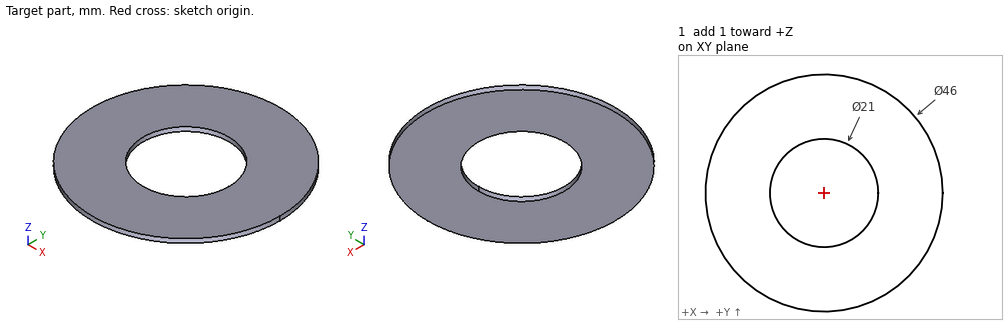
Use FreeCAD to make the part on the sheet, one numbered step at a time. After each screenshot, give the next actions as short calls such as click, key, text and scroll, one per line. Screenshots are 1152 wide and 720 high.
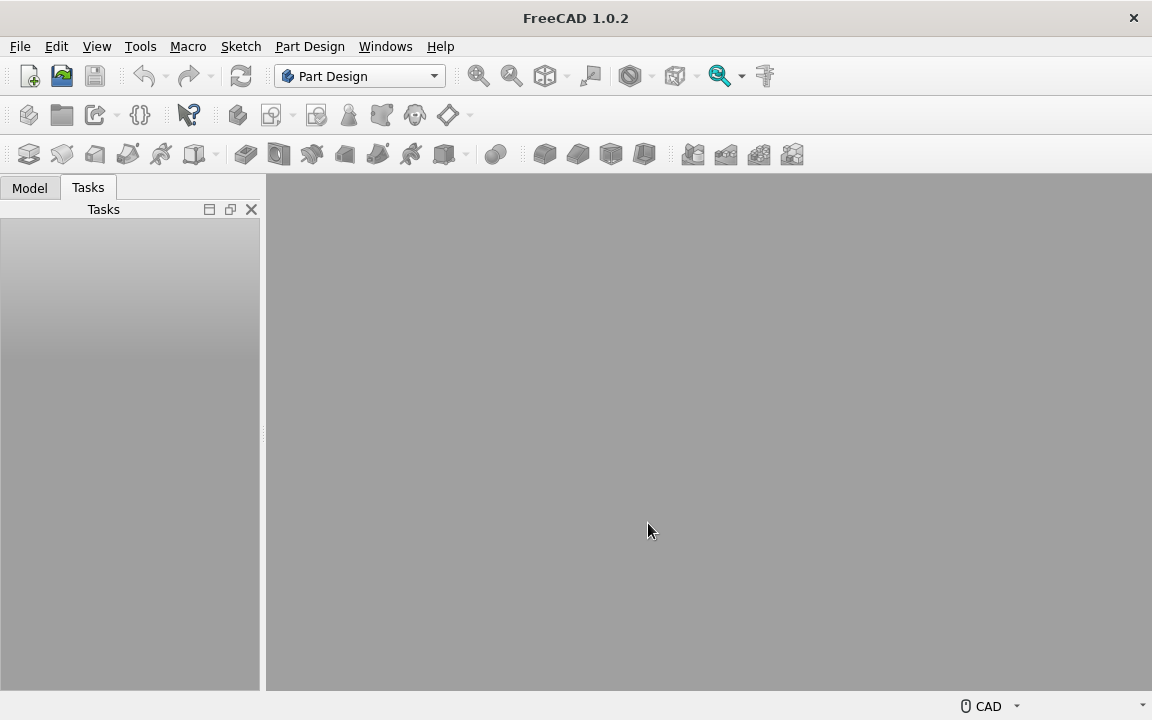
key(ctrl+n)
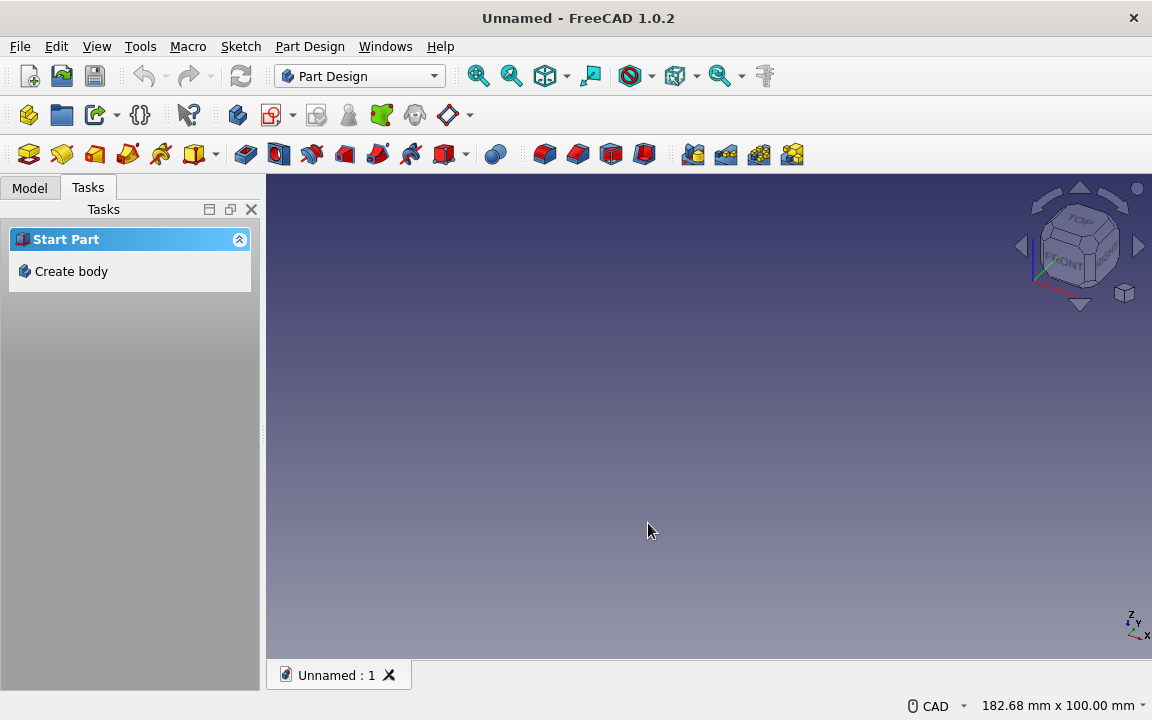
click(270, 116)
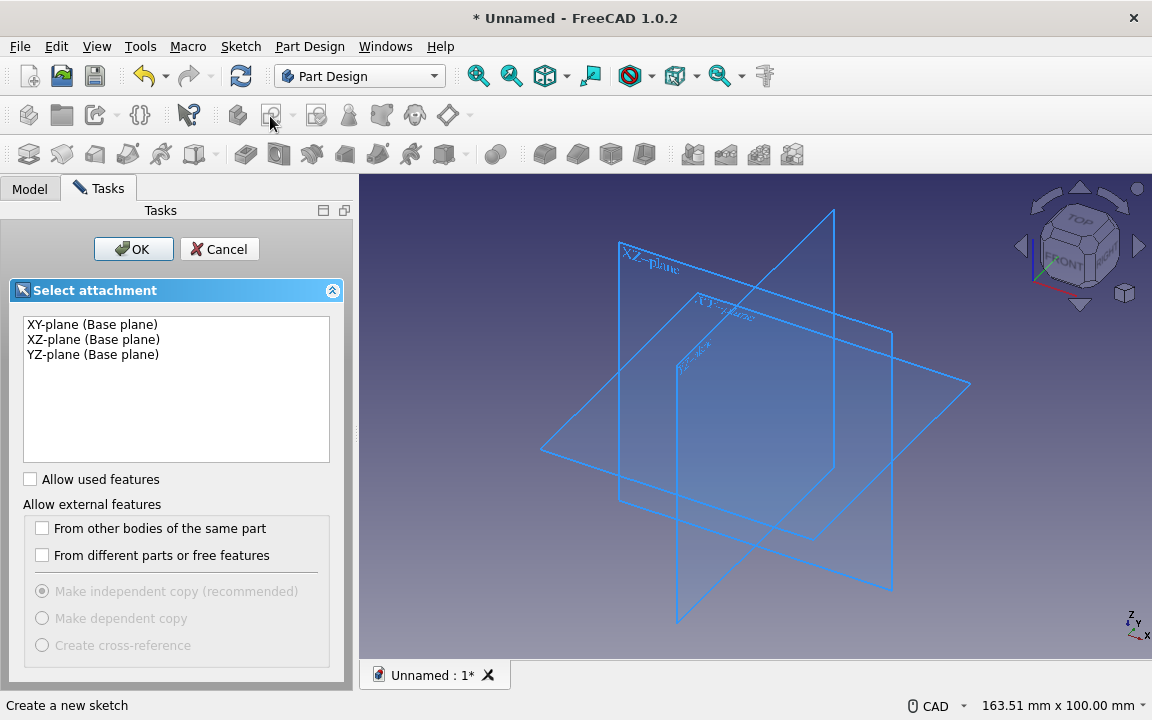
click(84, 324)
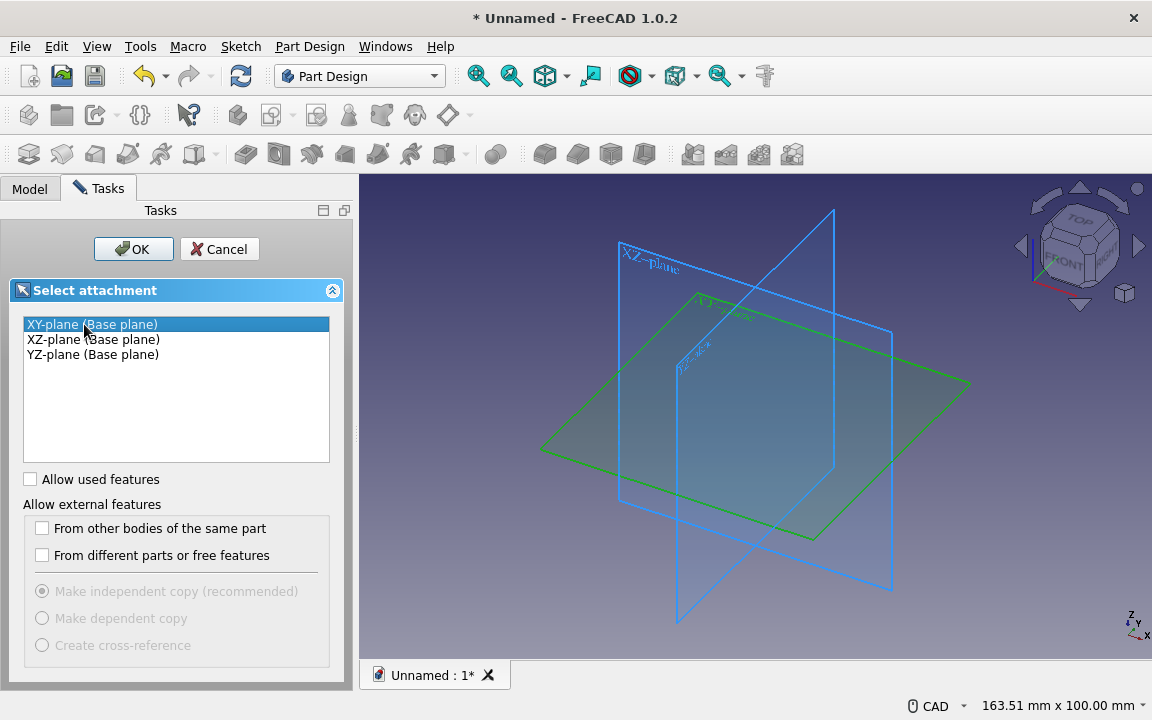
click(134, 249)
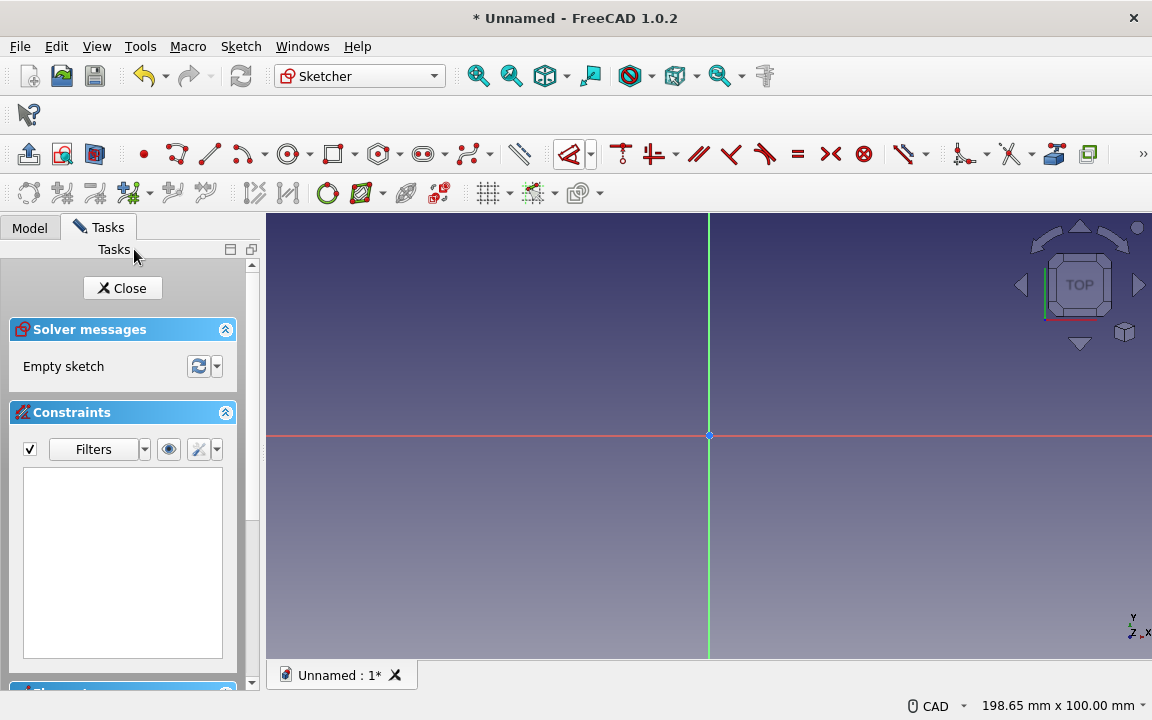
key(g)
key(c)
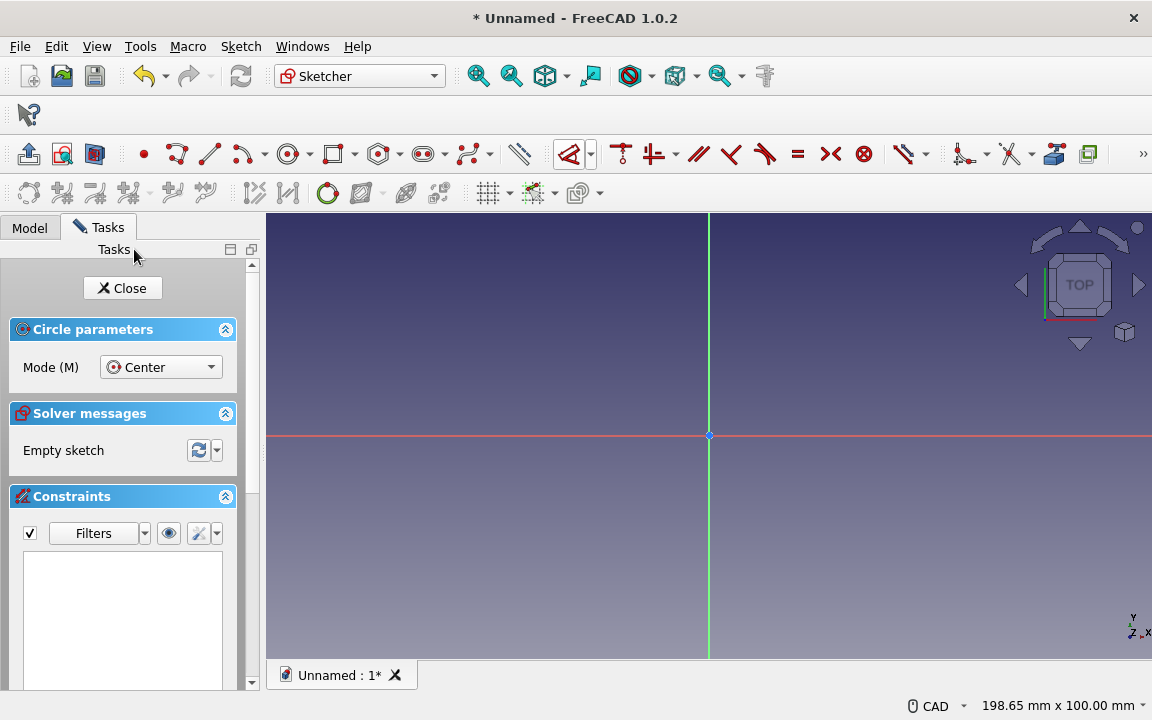
click(709, 436)
click(782, 363)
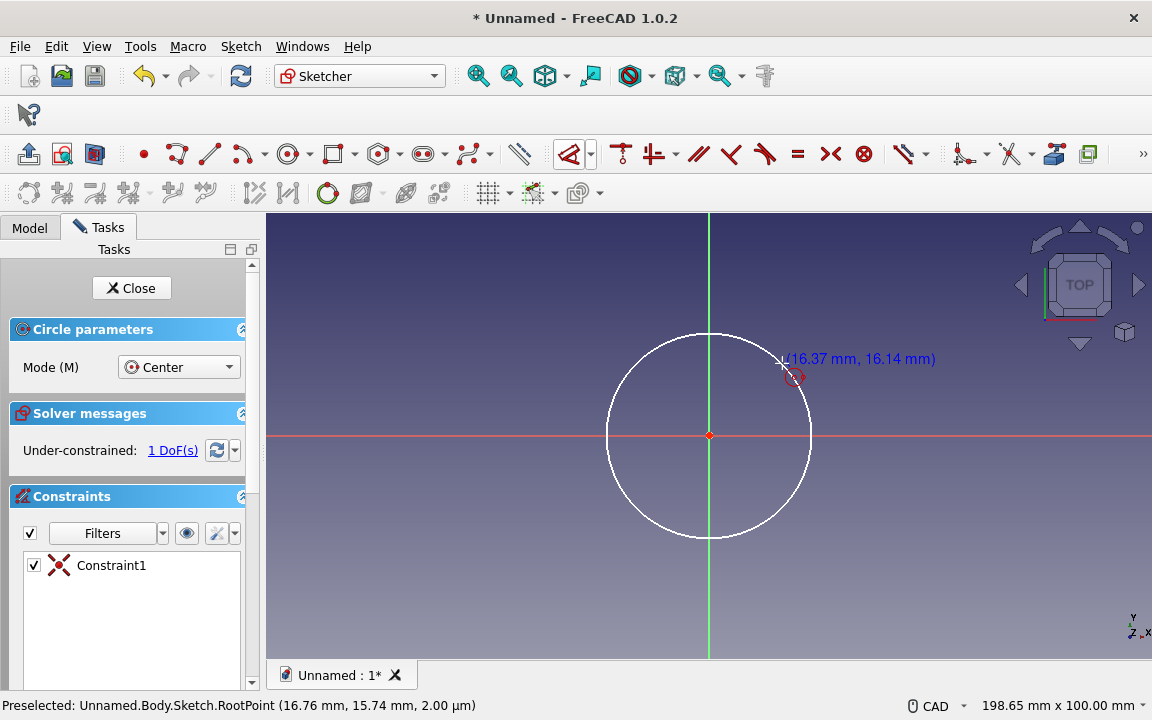
click(709, 436)
click(742, 403)
key(Escape)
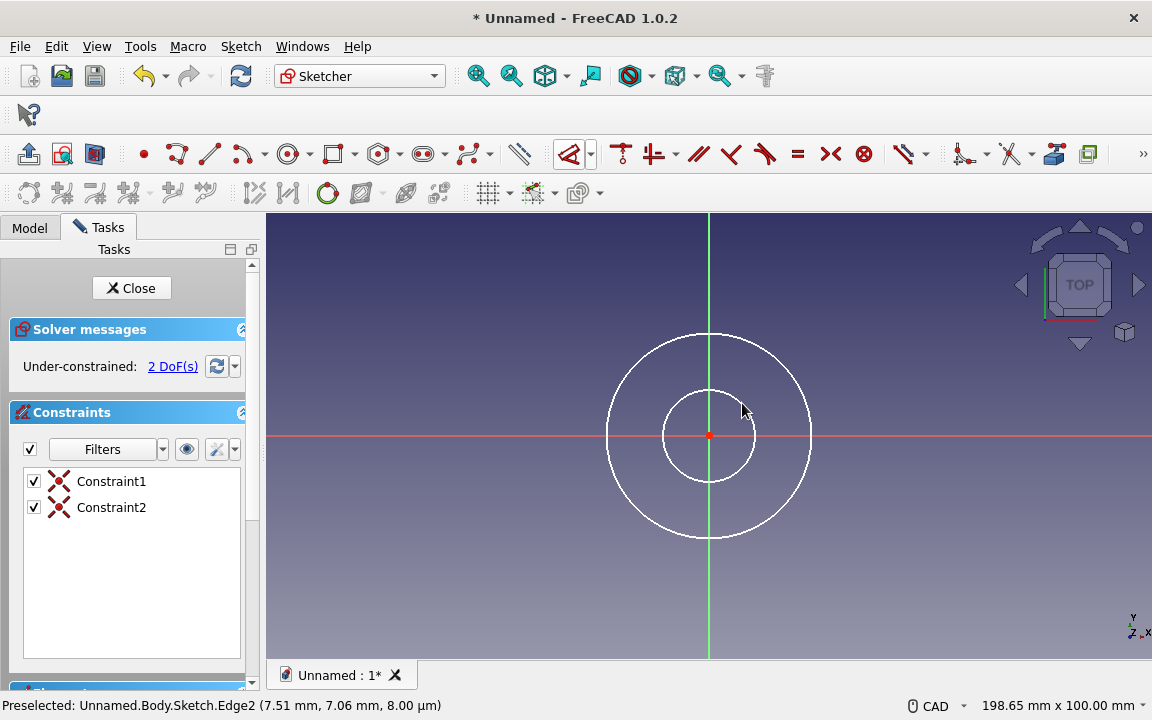
key(d)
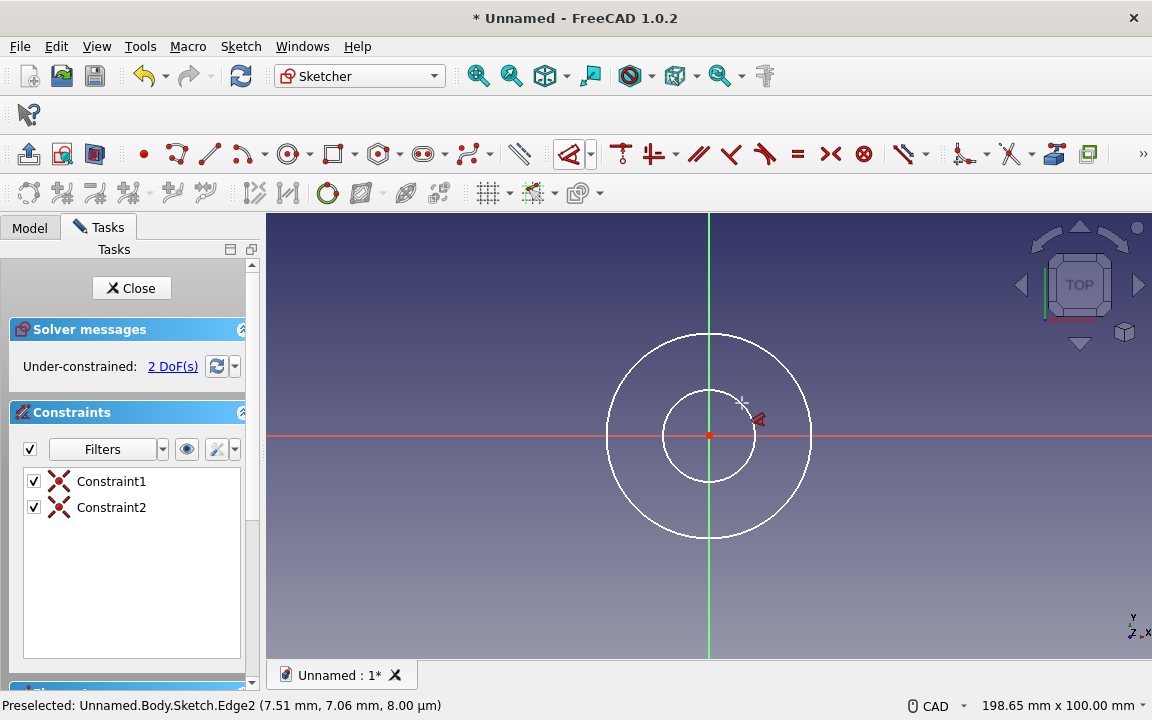
click(781, 363)
click(803, 340)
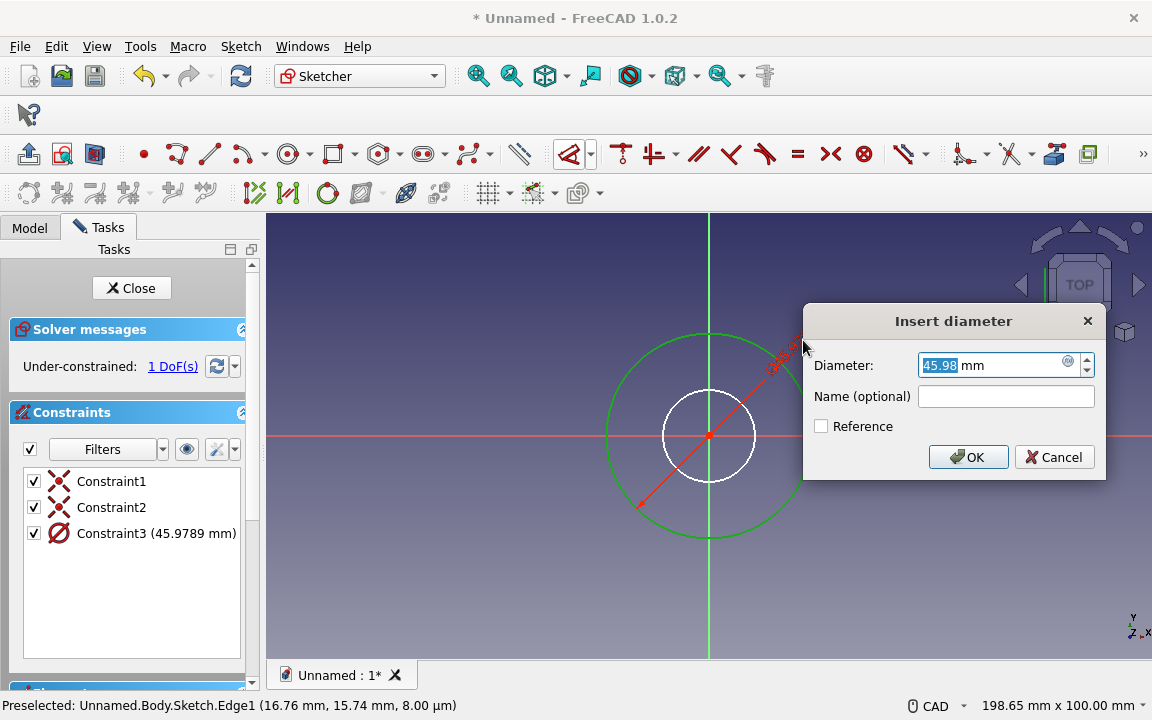
text(46)
key(Return)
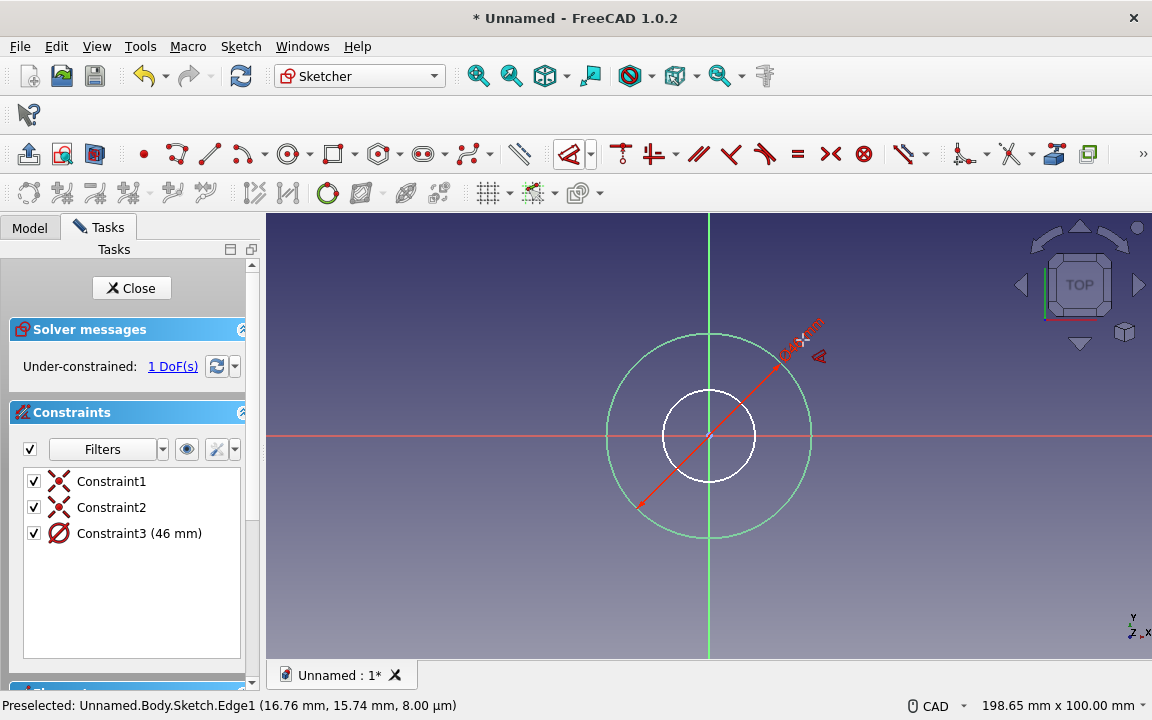
click(741, 403)
click(763, 380)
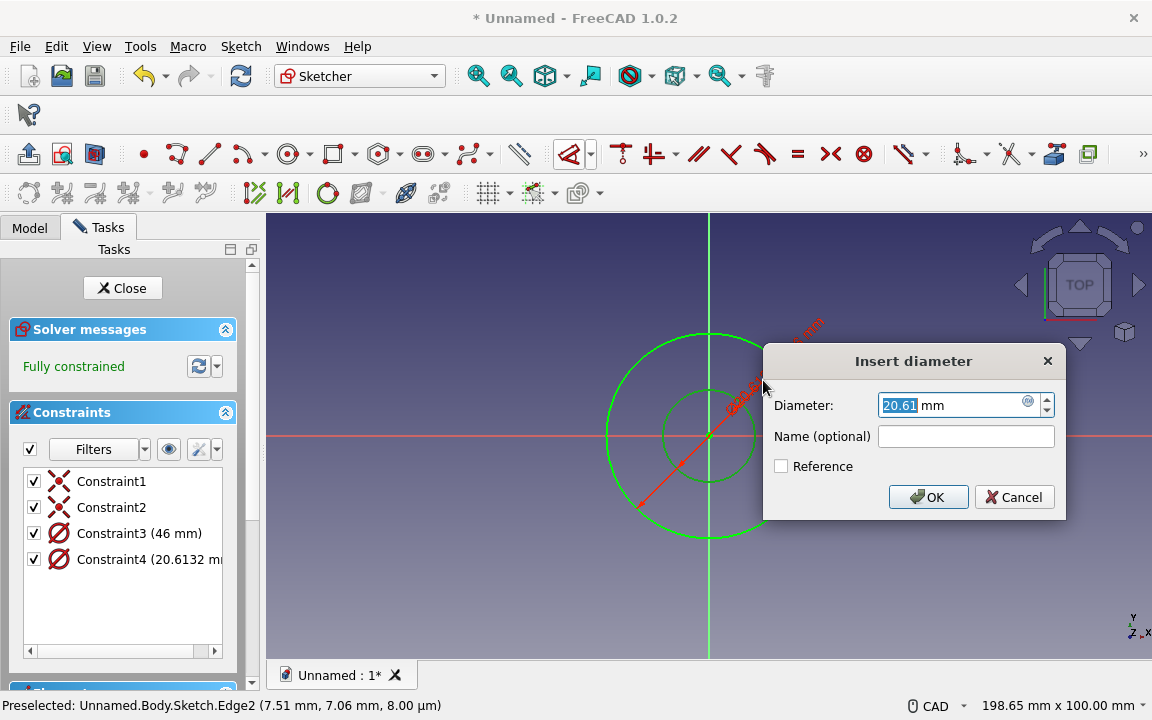
text(21)
key(Return)
key(Escape)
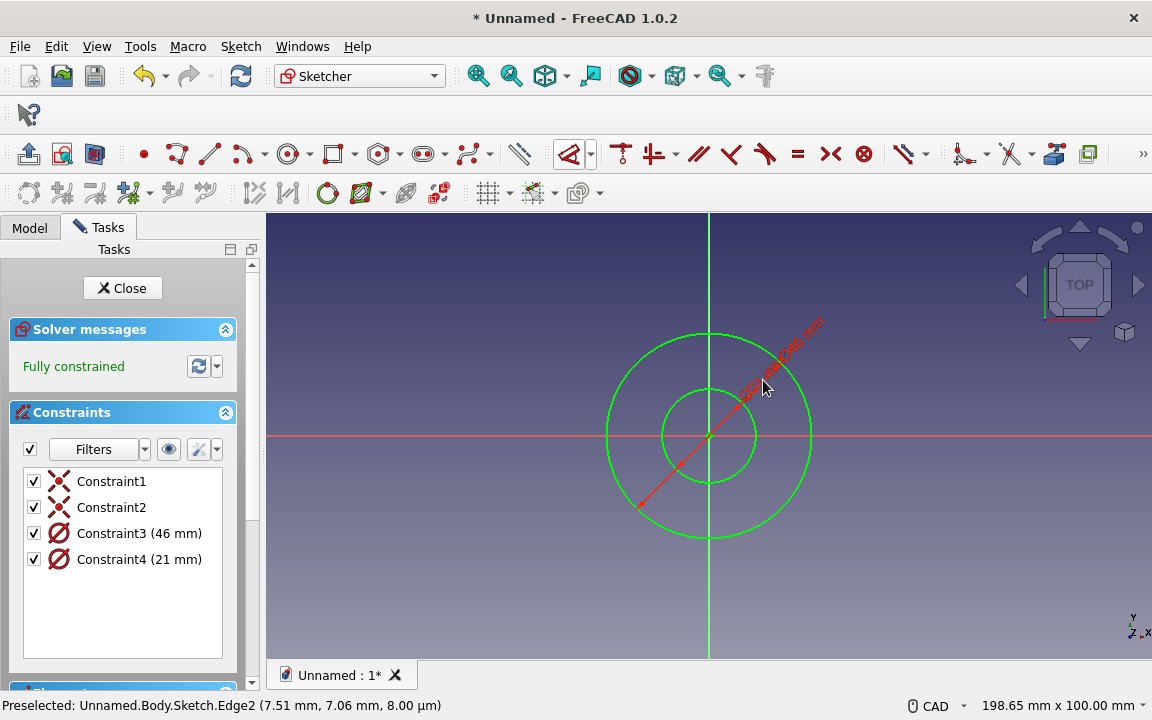
click(123, 288)